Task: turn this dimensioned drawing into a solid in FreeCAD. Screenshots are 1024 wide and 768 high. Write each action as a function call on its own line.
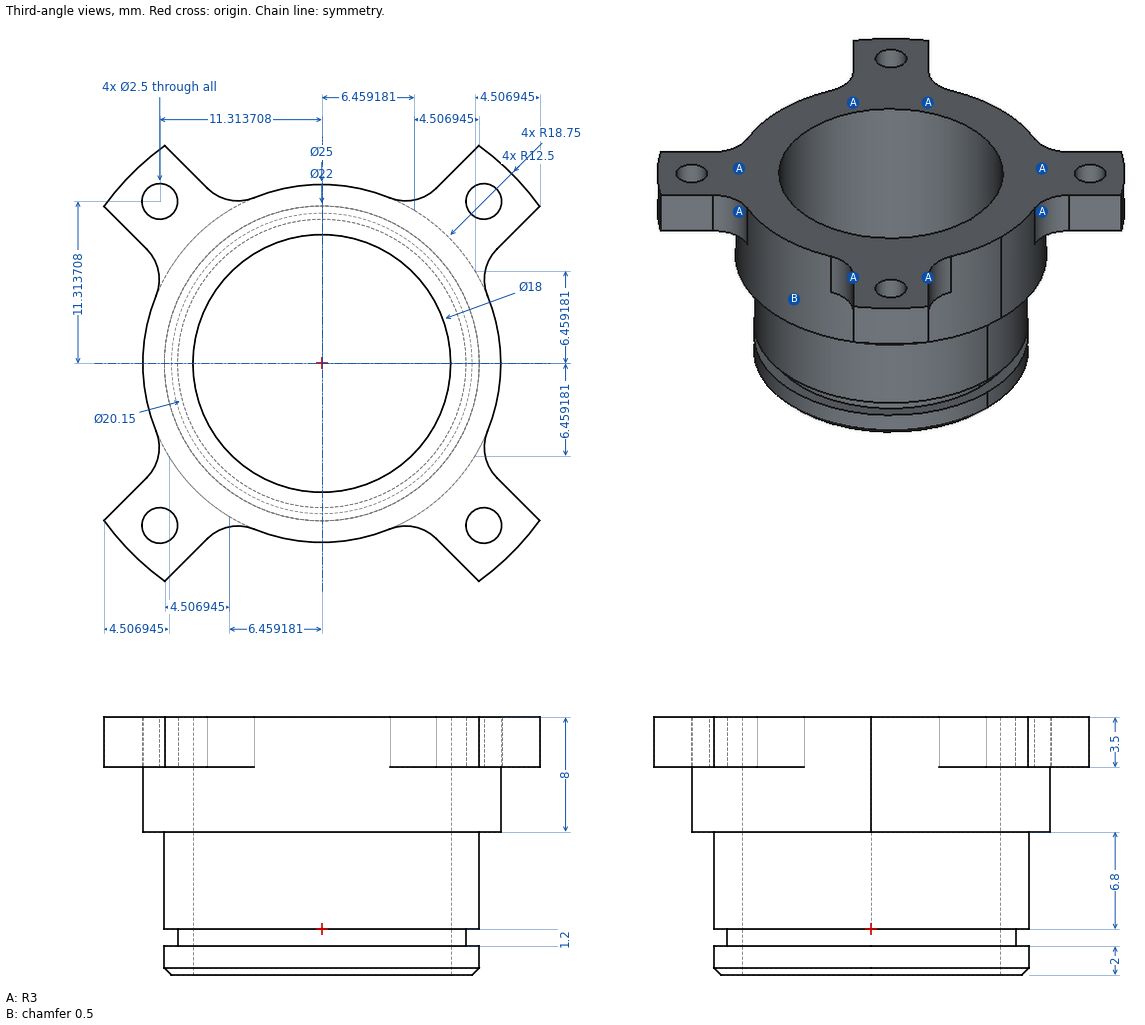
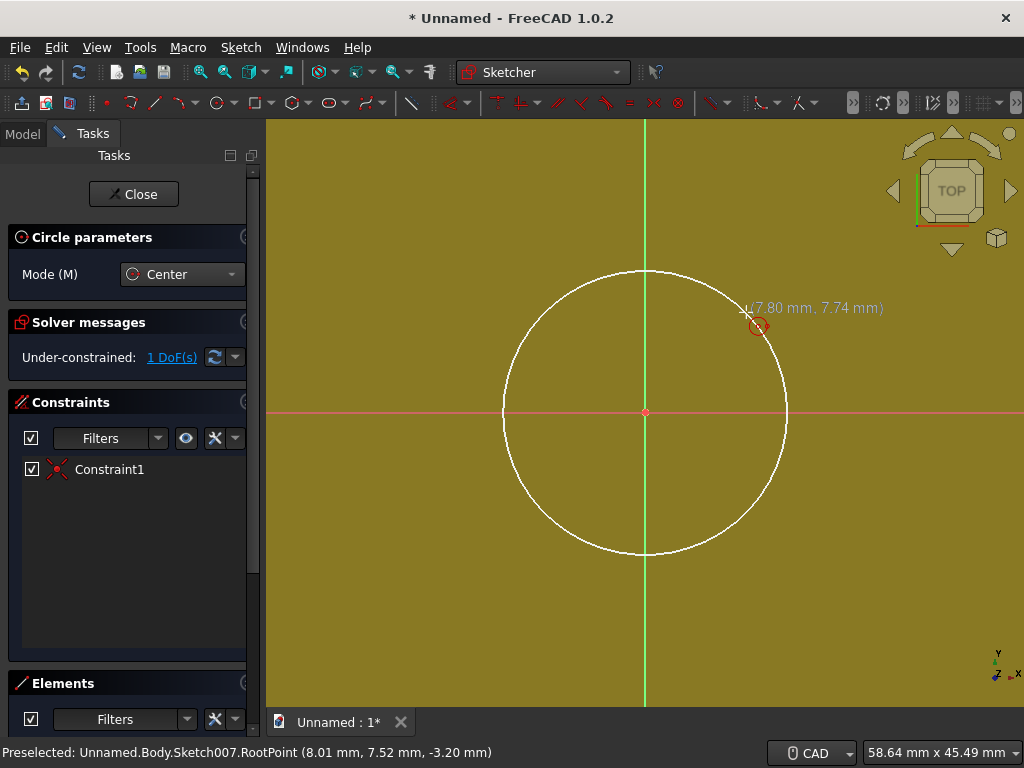
click(645, 413)
click(727, 331)
key(Escape)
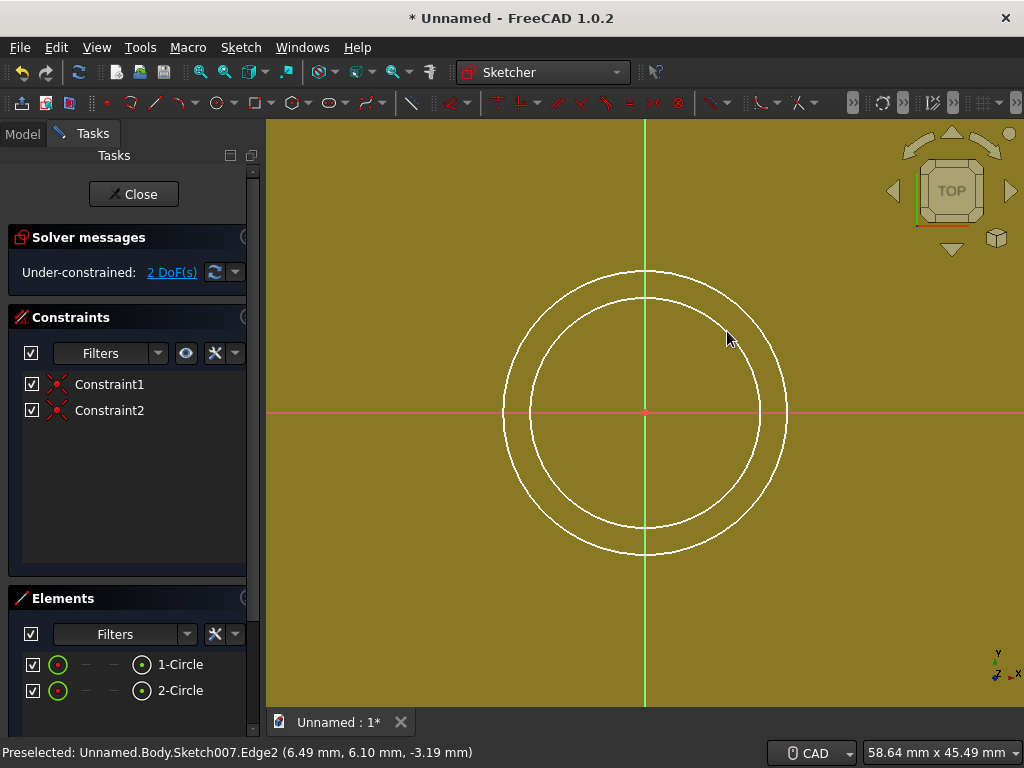
click(450, 104)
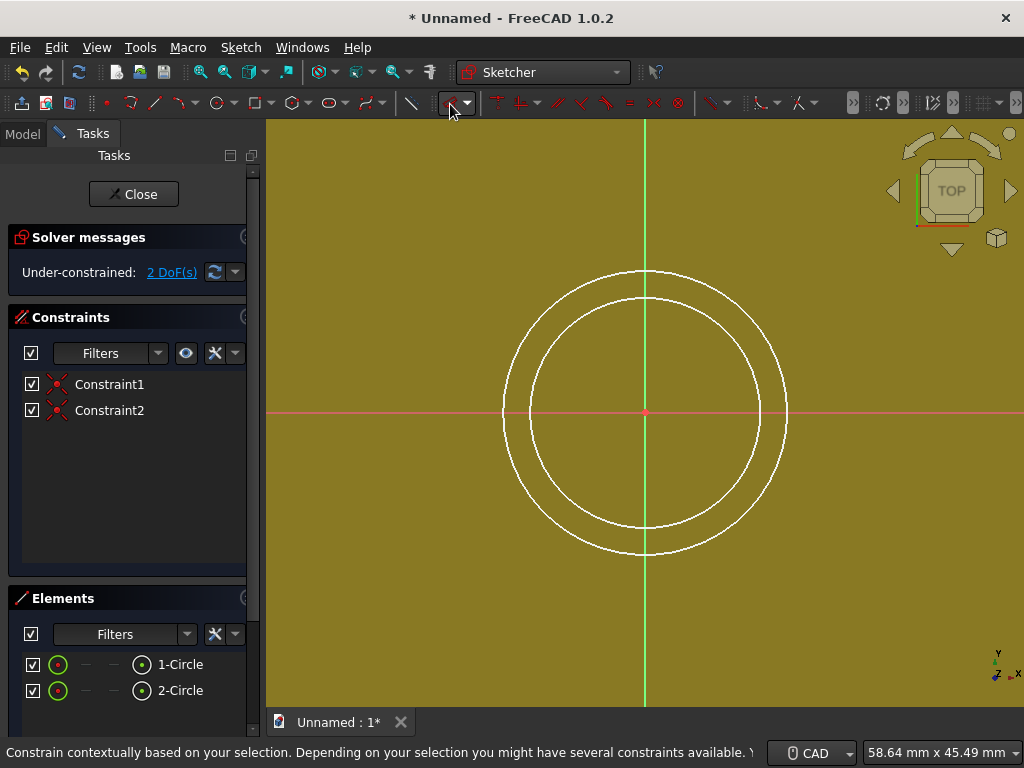
click(745, 312)
click(767, 289)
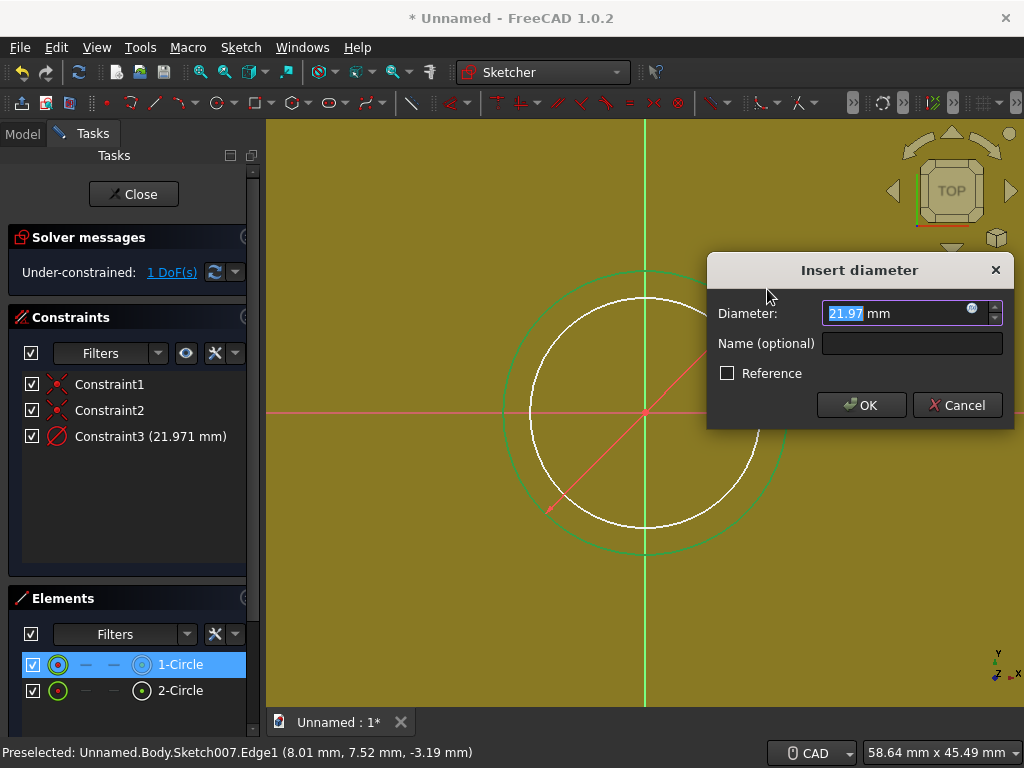
text(22)
key(Return)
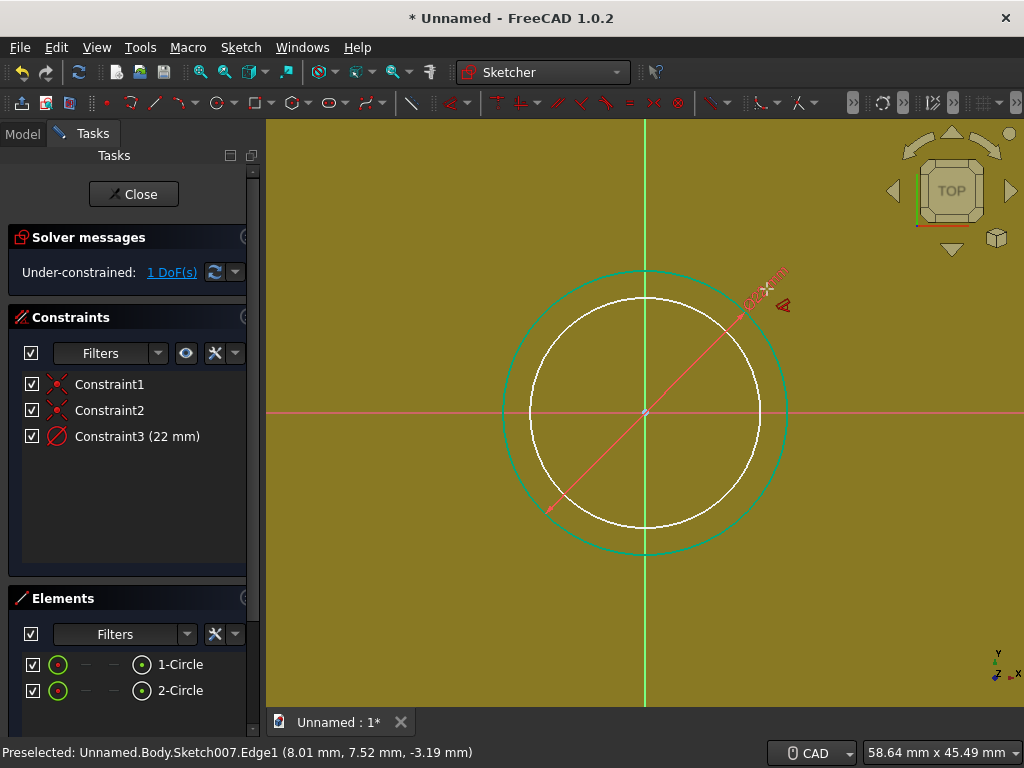
click(726, 331)
click(808, 364)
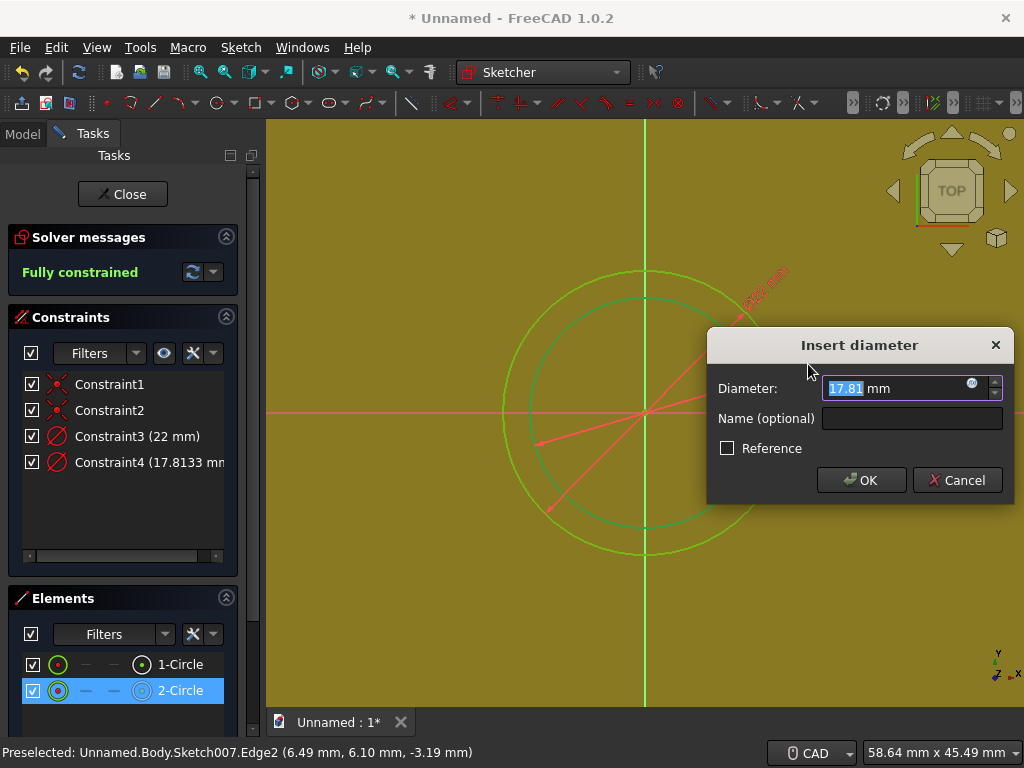
text(18)
key(Return)
key(Escape)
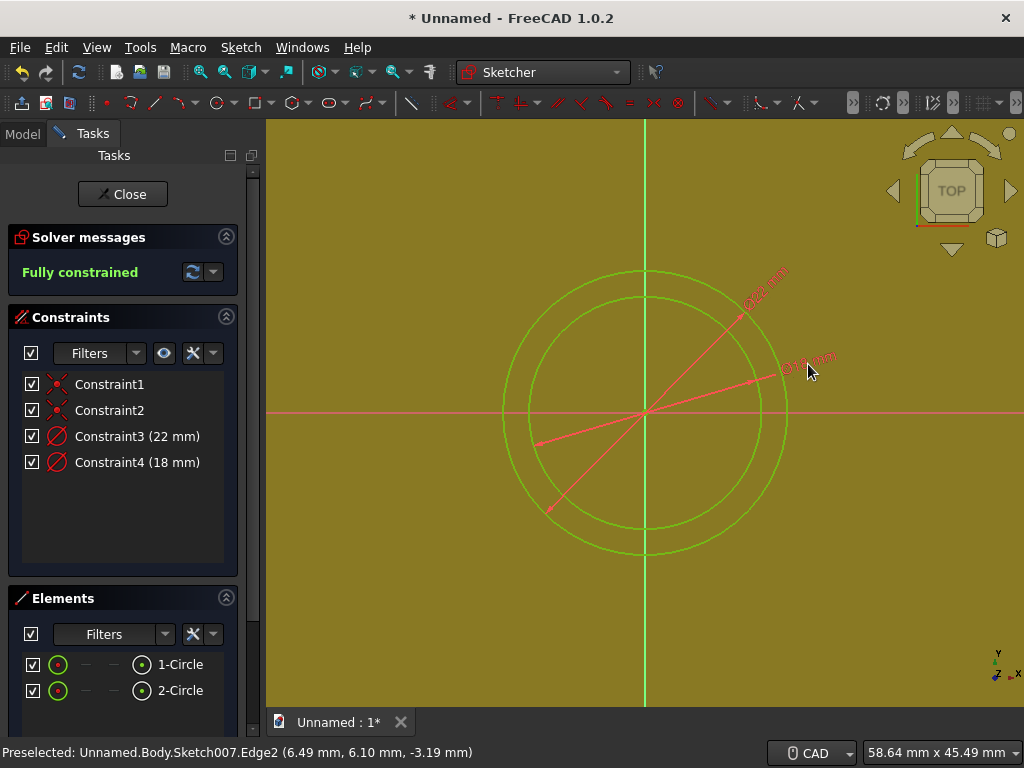
click(123, 194)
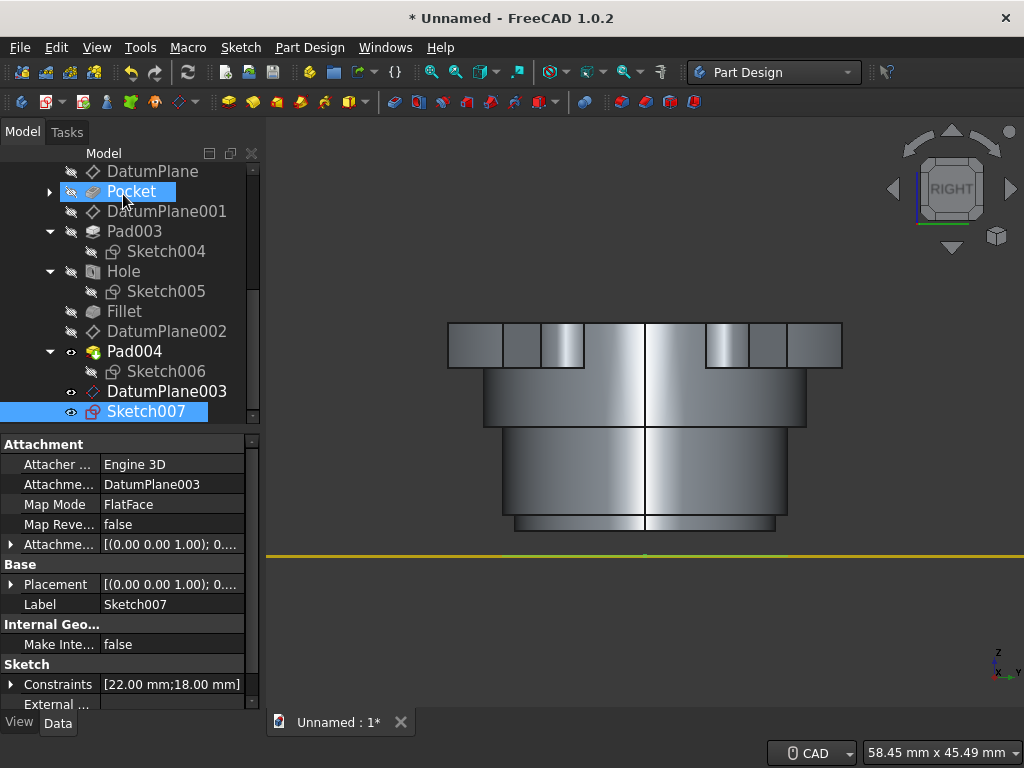
click(230, 102)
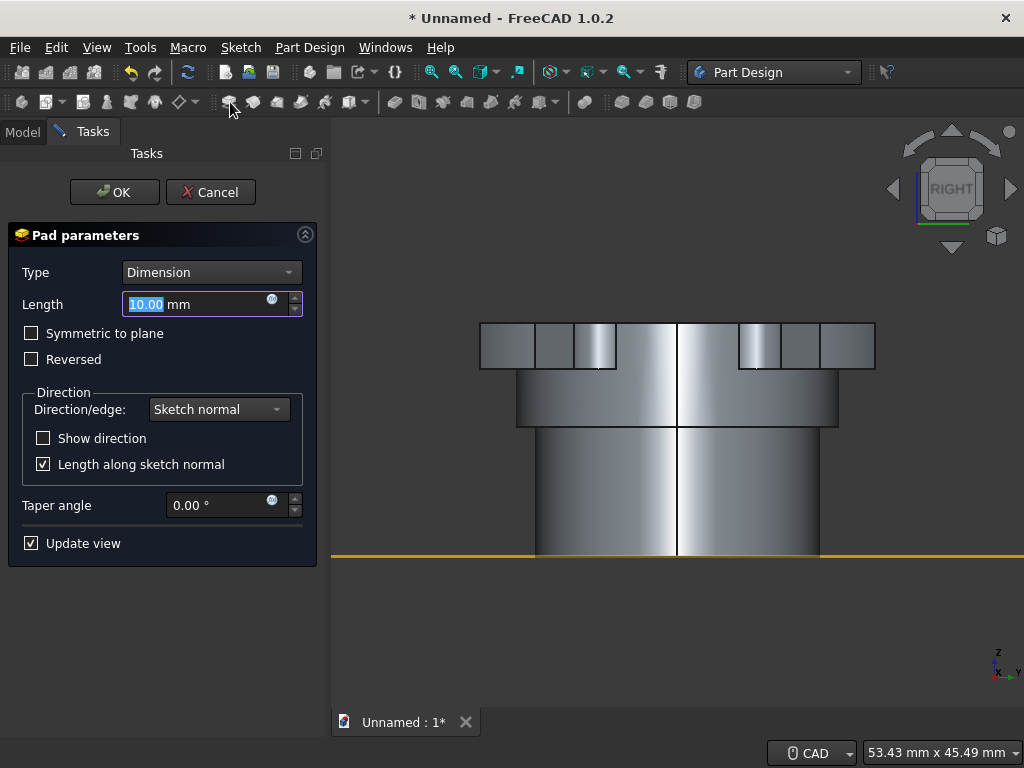
text(2)
key(Tab)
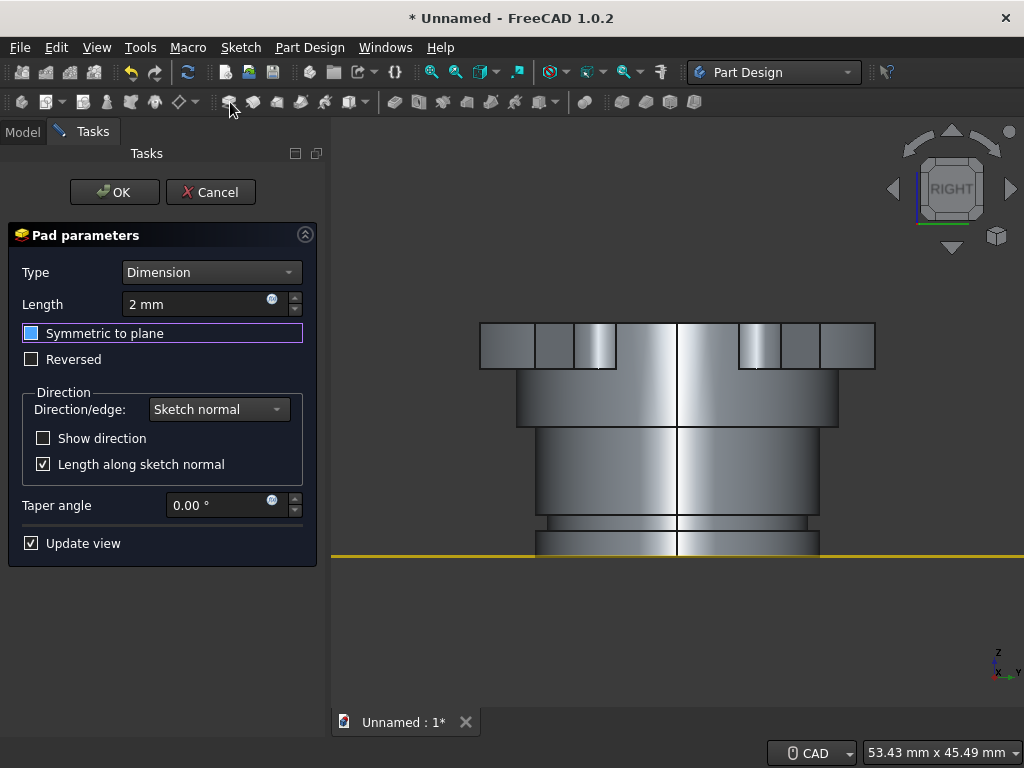
click(115, 192)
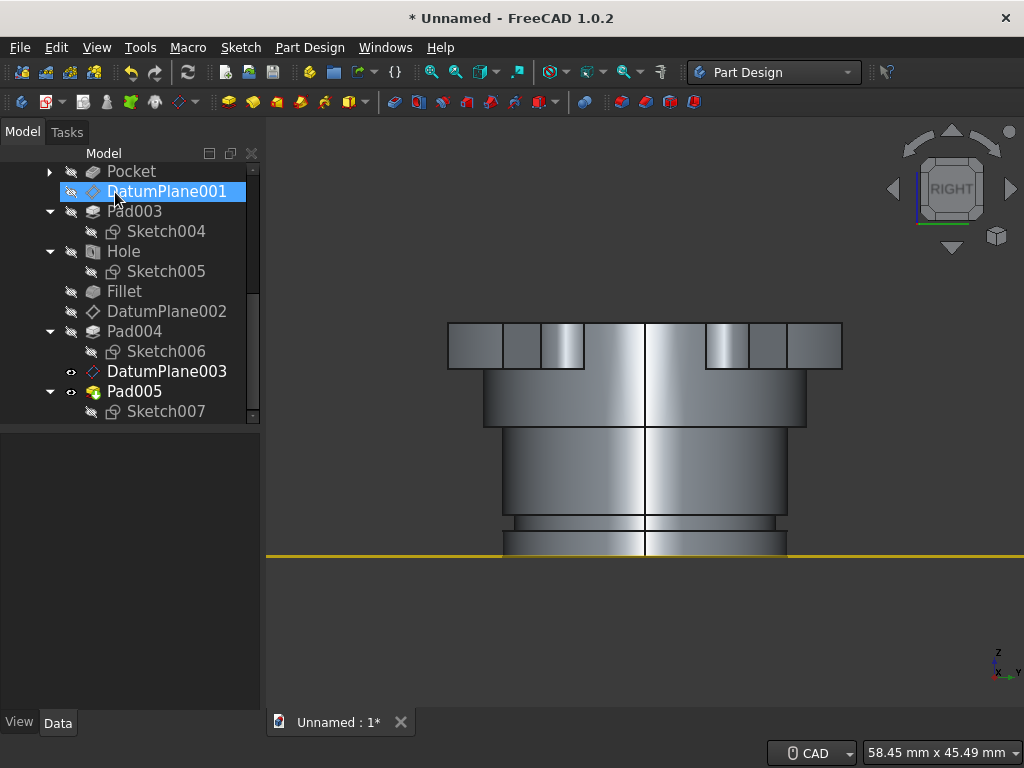
click(116, 372)
key(space)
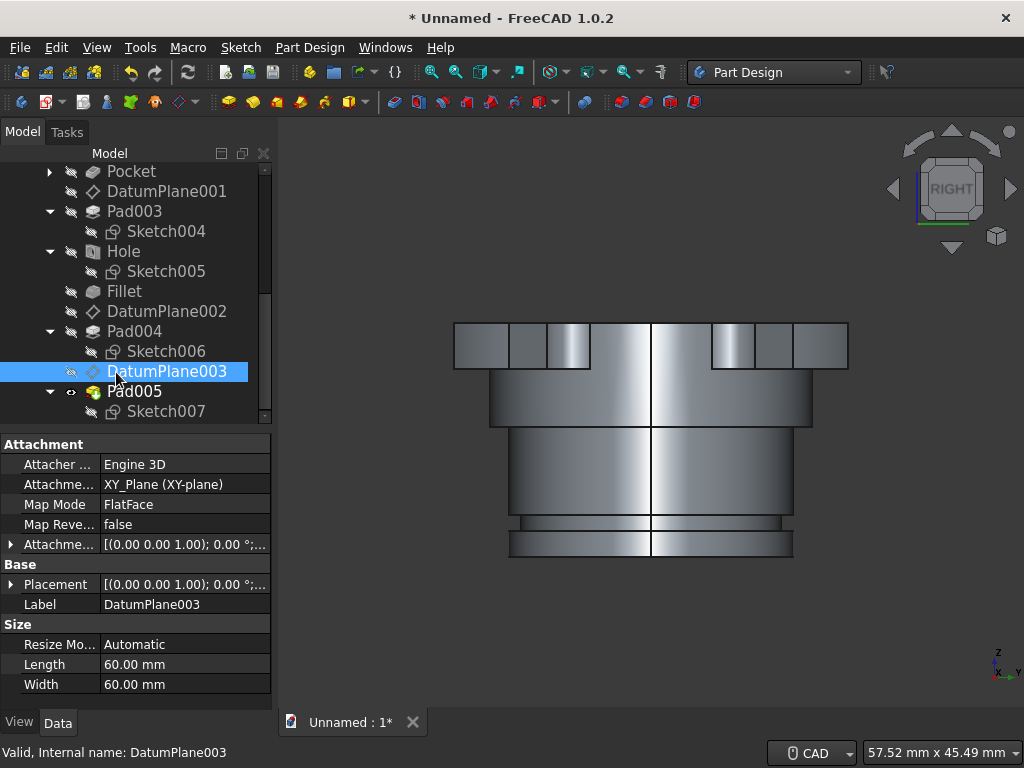
click(735, 556)